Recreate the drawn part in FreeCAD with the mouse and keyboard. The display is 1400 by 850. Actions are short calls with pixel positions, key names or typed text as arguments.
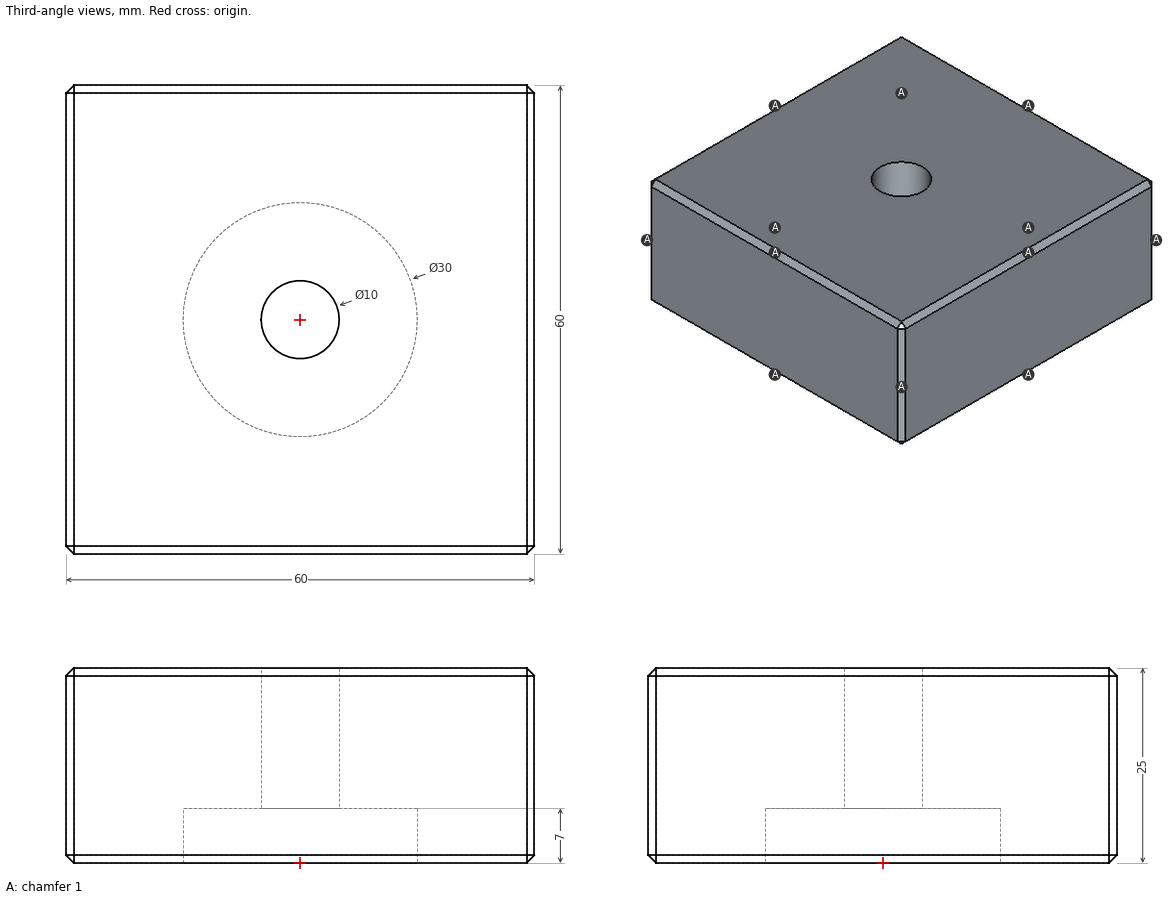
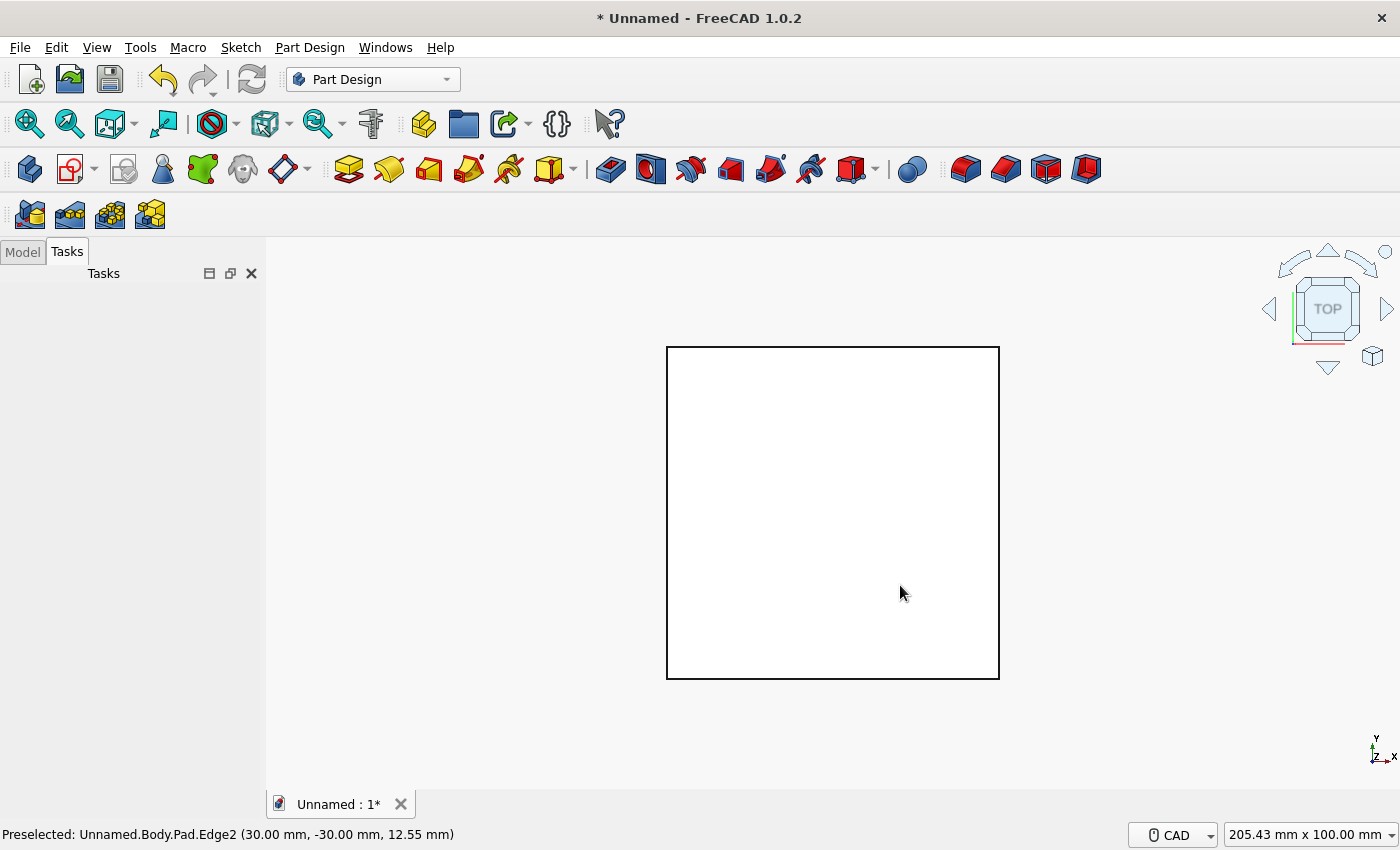
key(1)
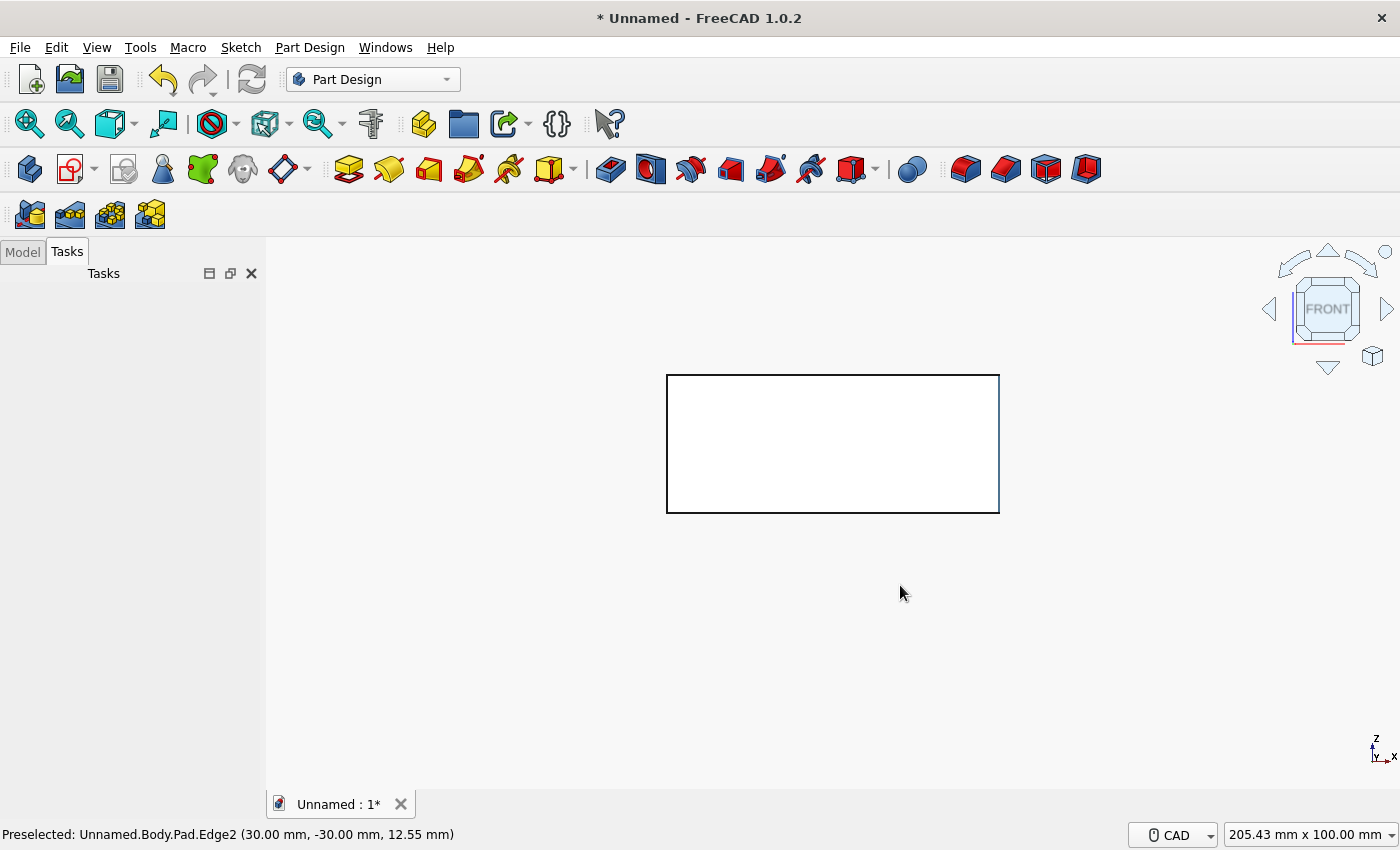
click(30, 124)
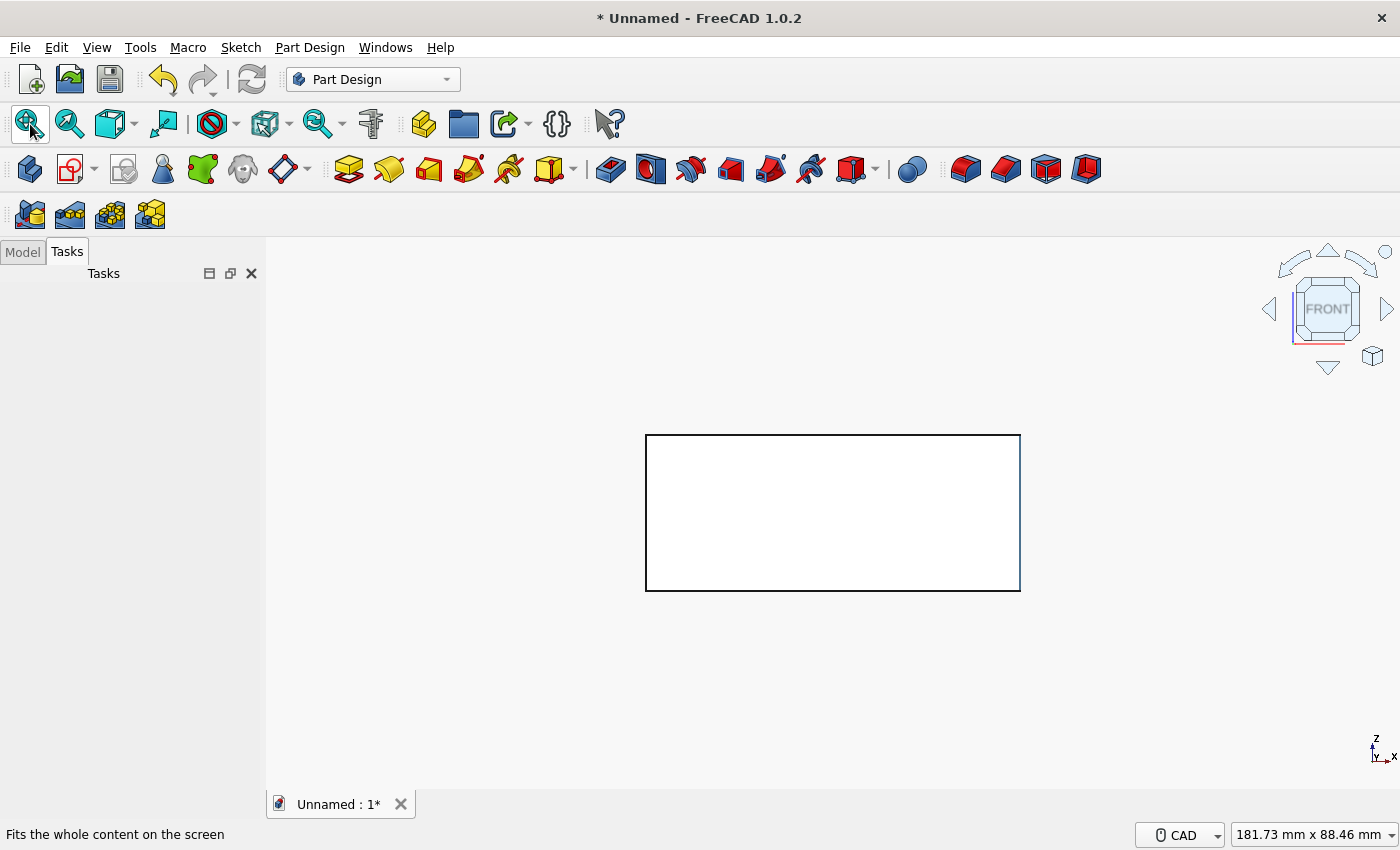
click(646, 512, ctrl)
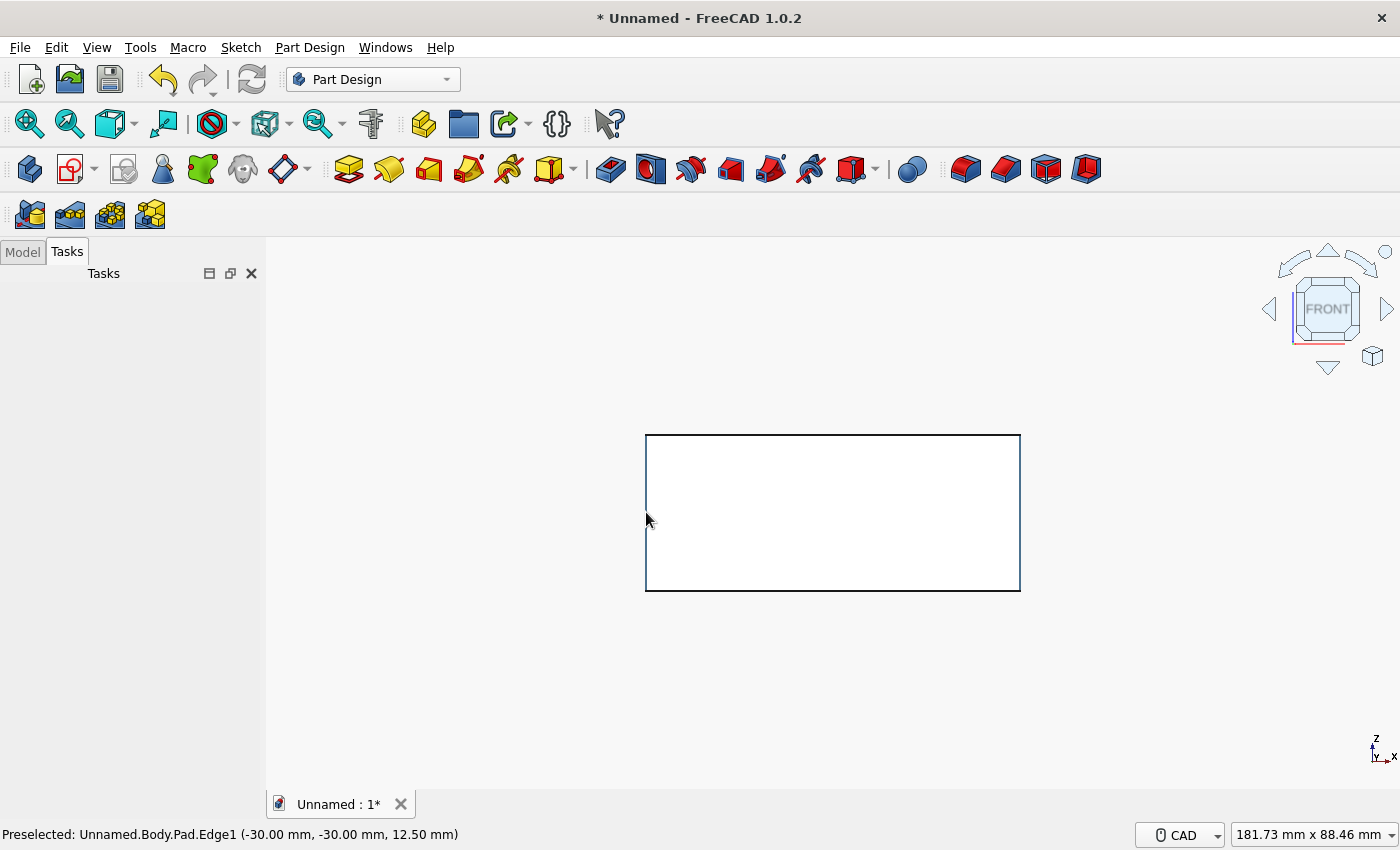
key(3)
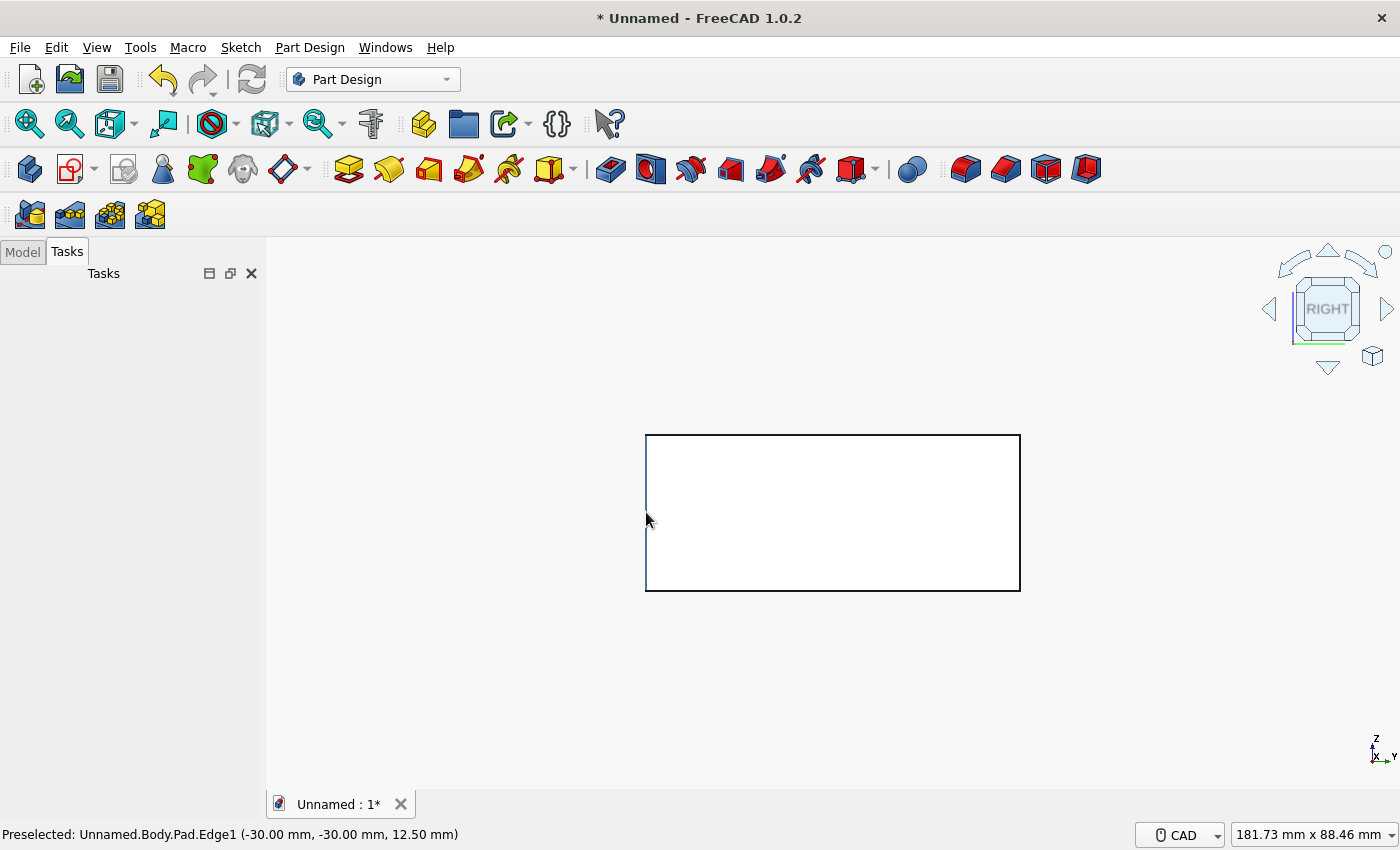
key(v)
key(f)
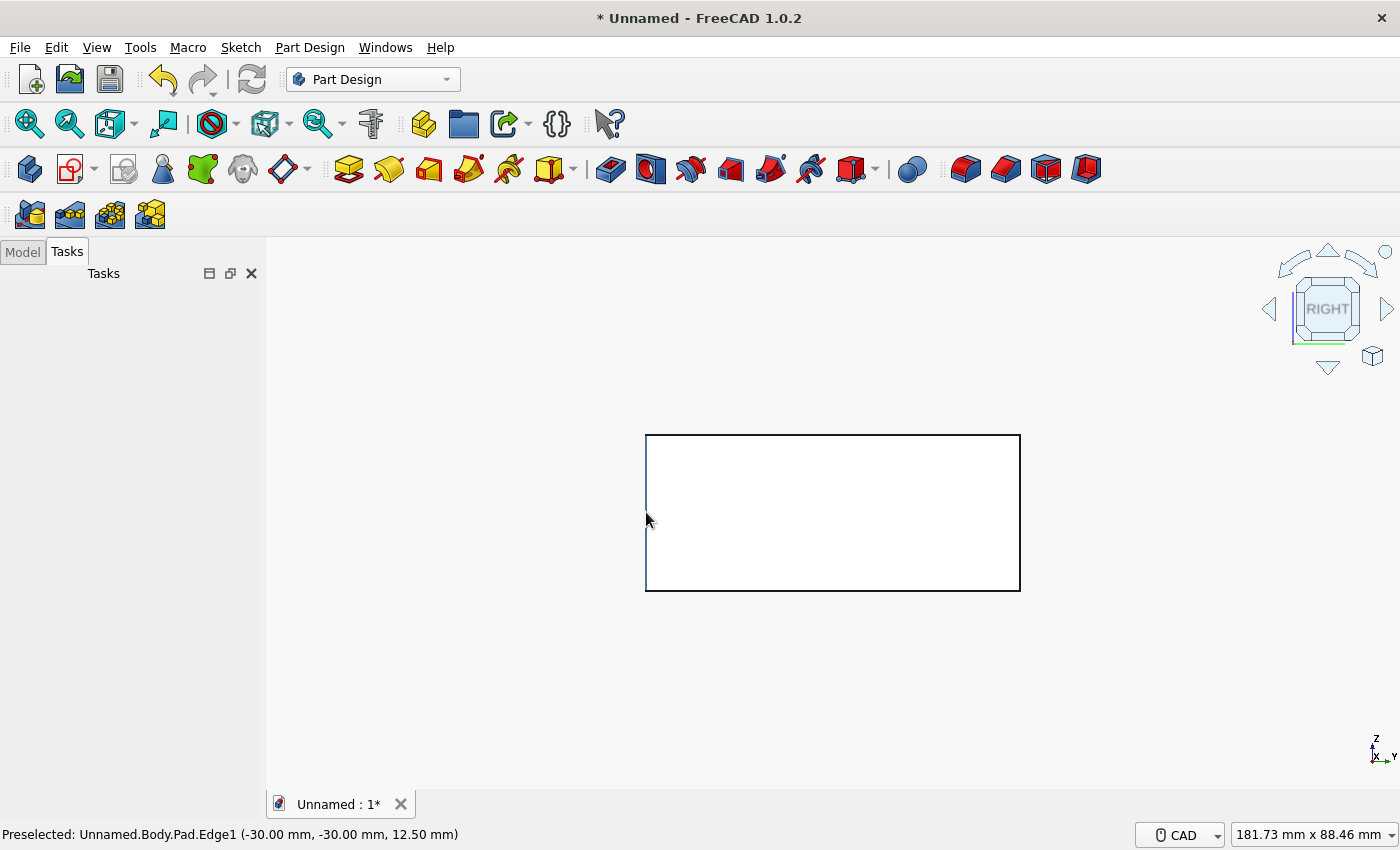
click(1020, 512, ctrl)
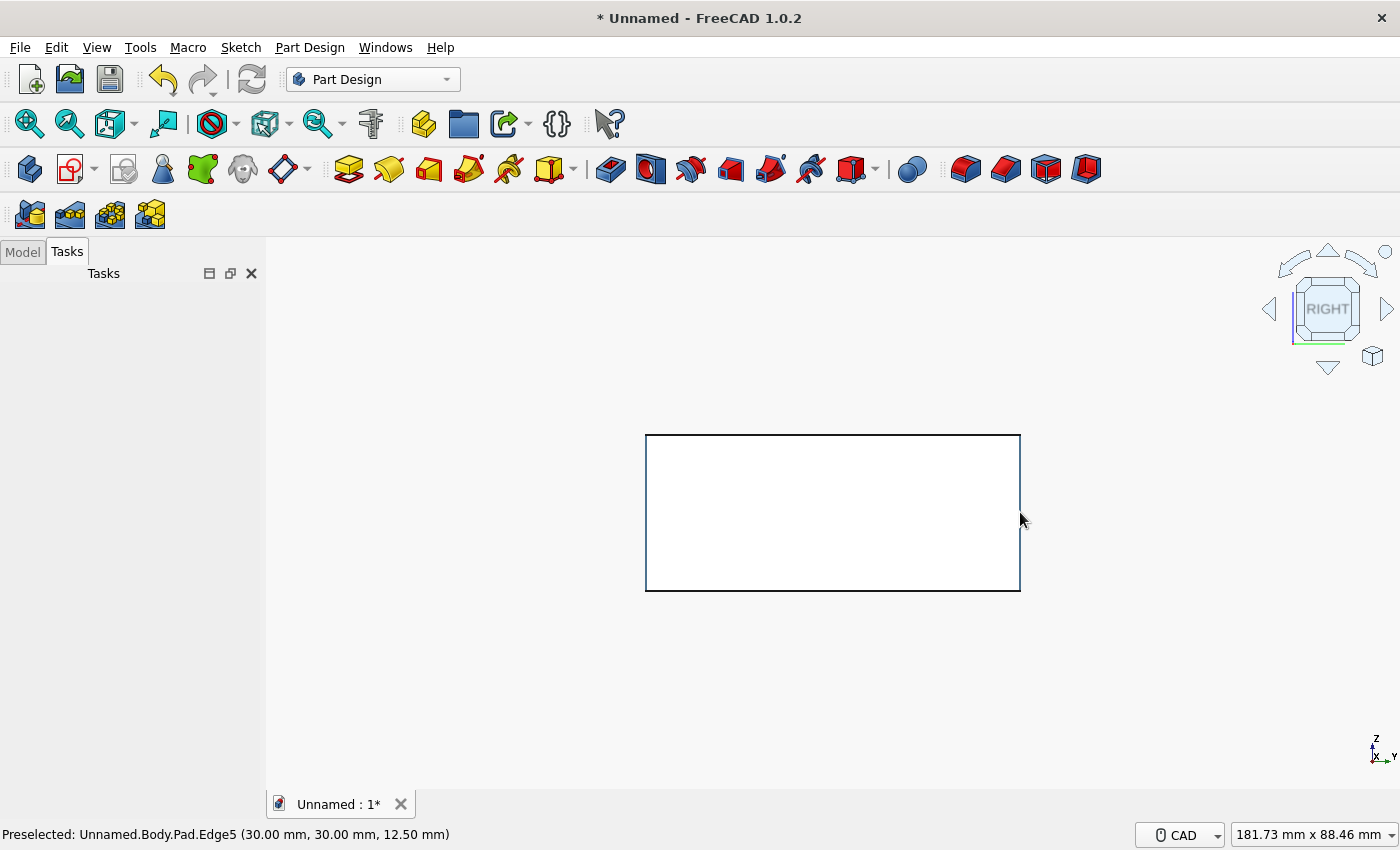
key(5)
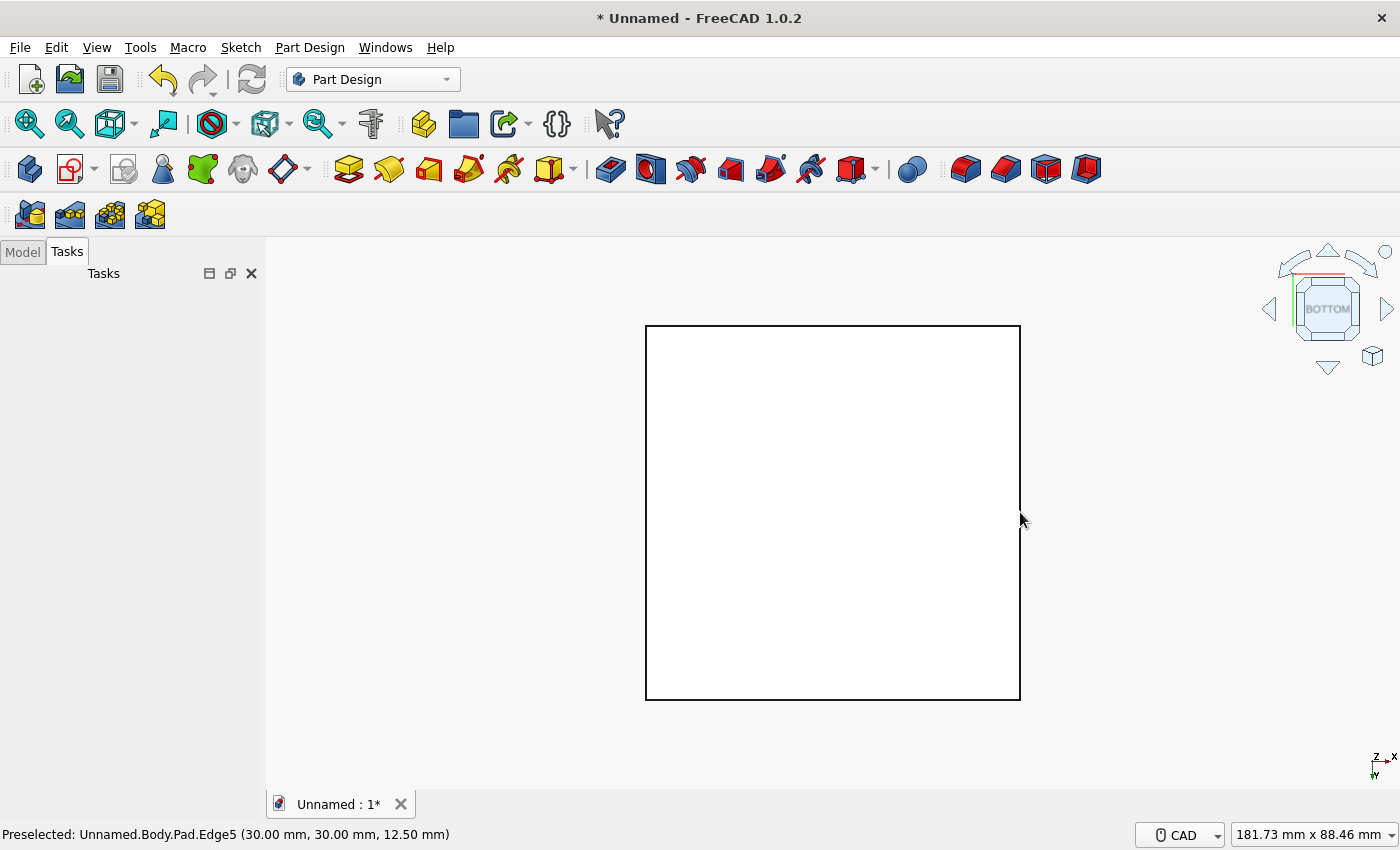
click(833, 512, ctrl)